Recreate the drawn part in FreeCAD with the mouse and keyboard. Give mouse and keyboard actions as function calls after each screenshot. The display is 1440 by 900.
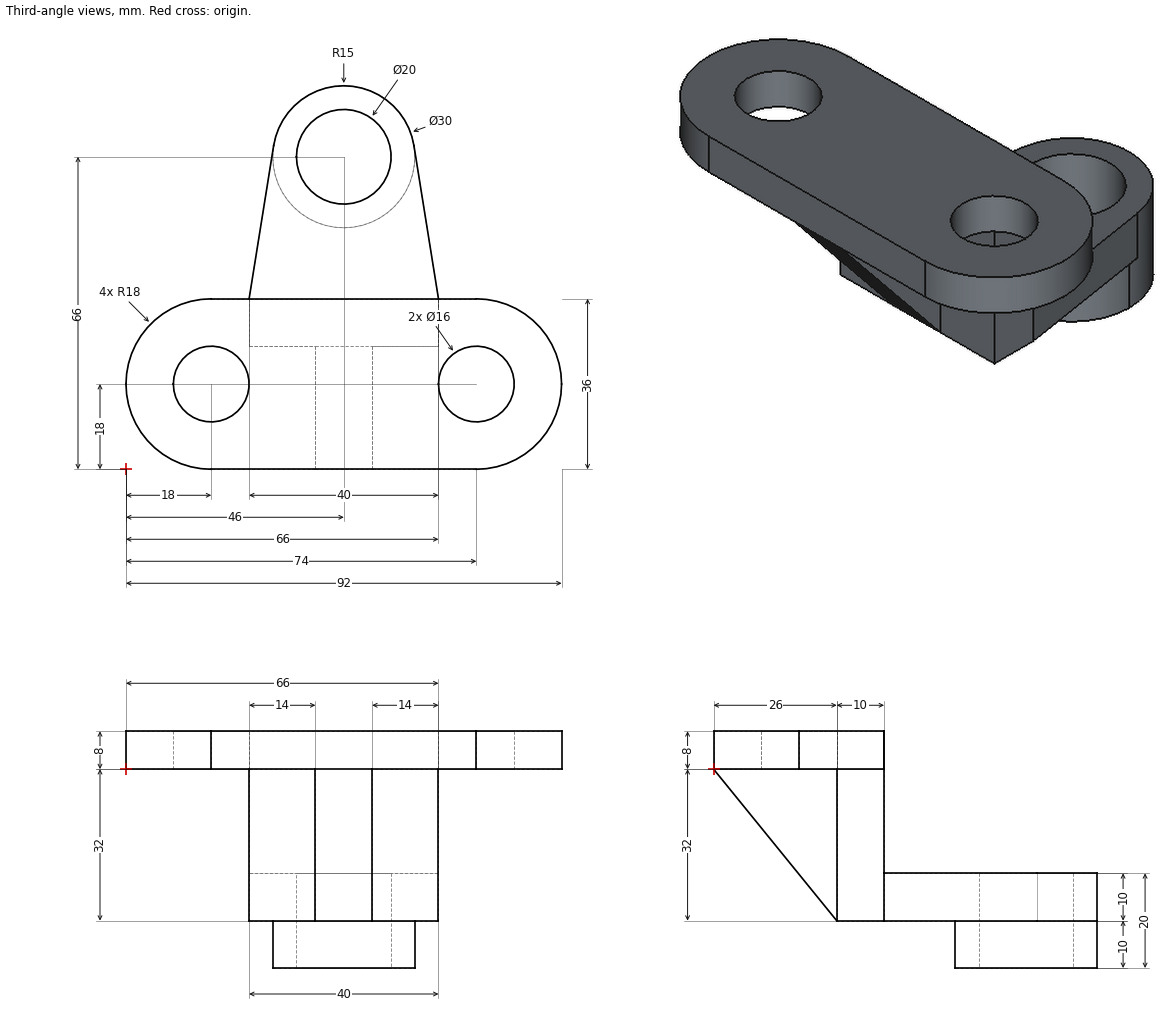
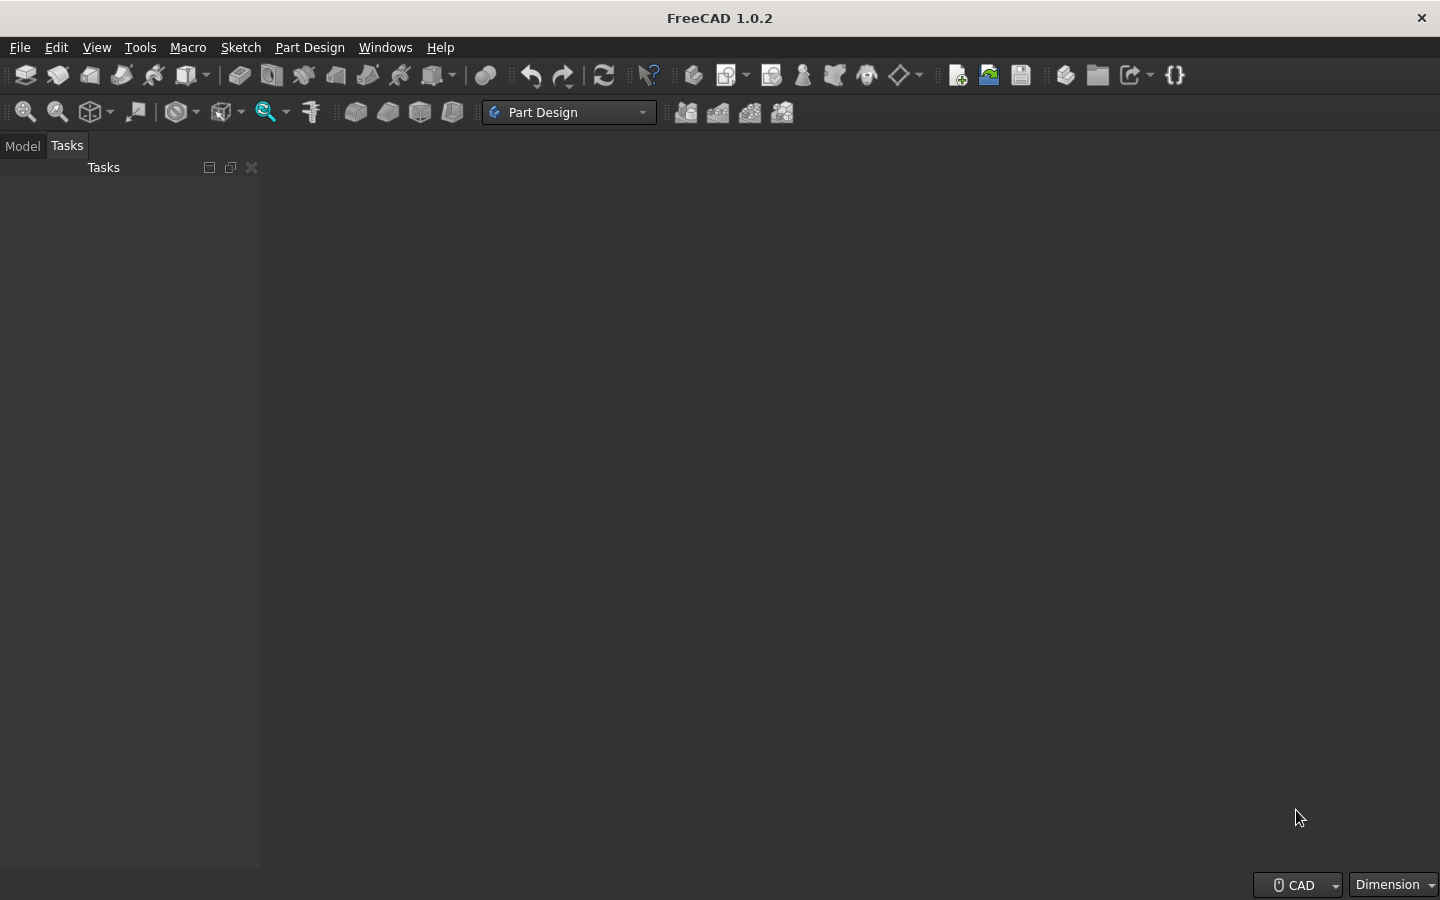
click(958, 76)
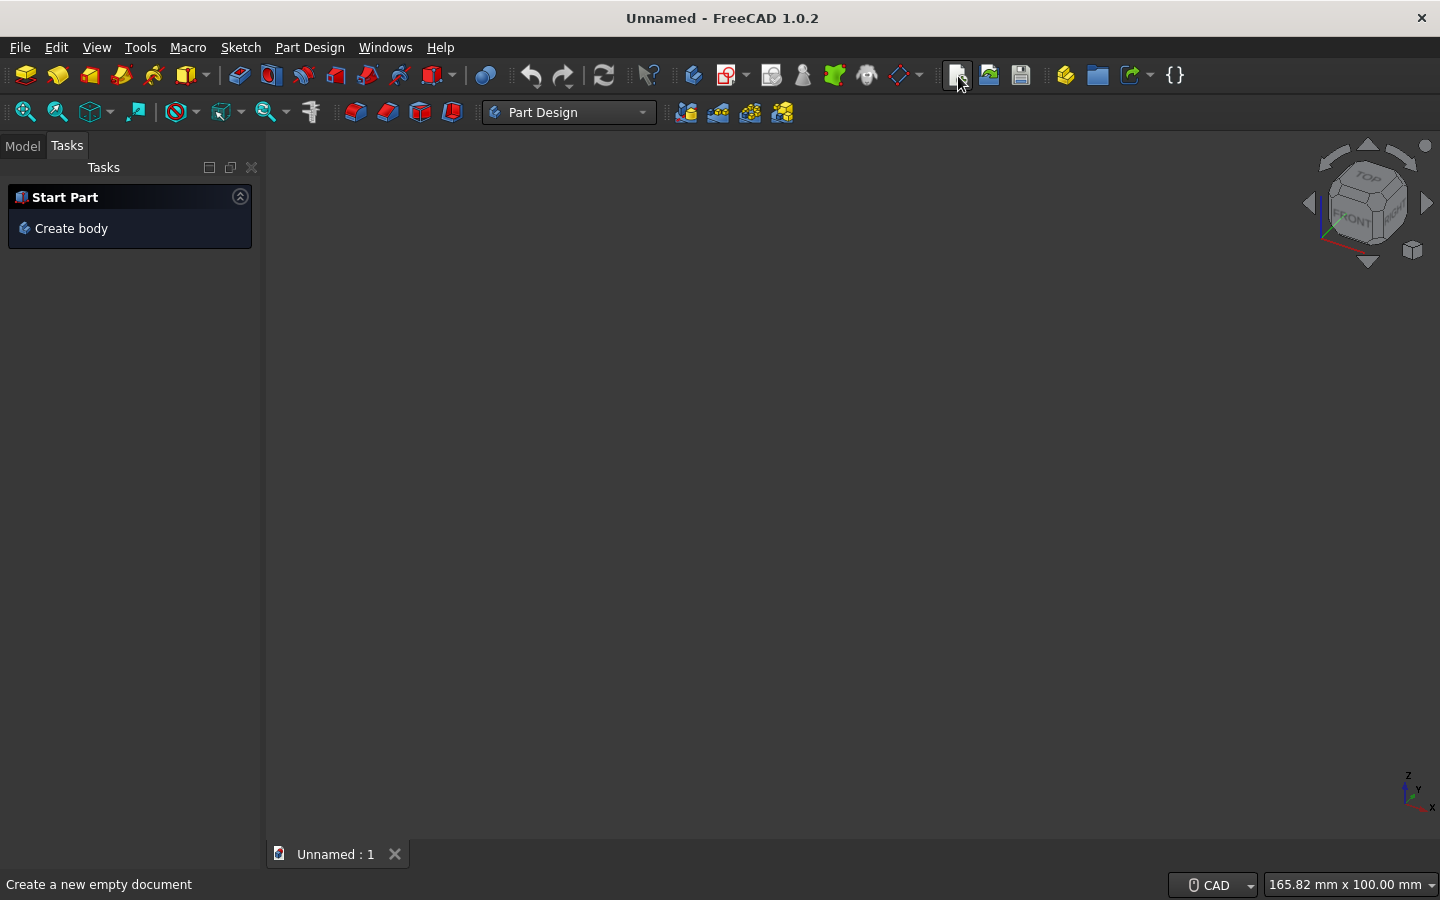
click(726, 76)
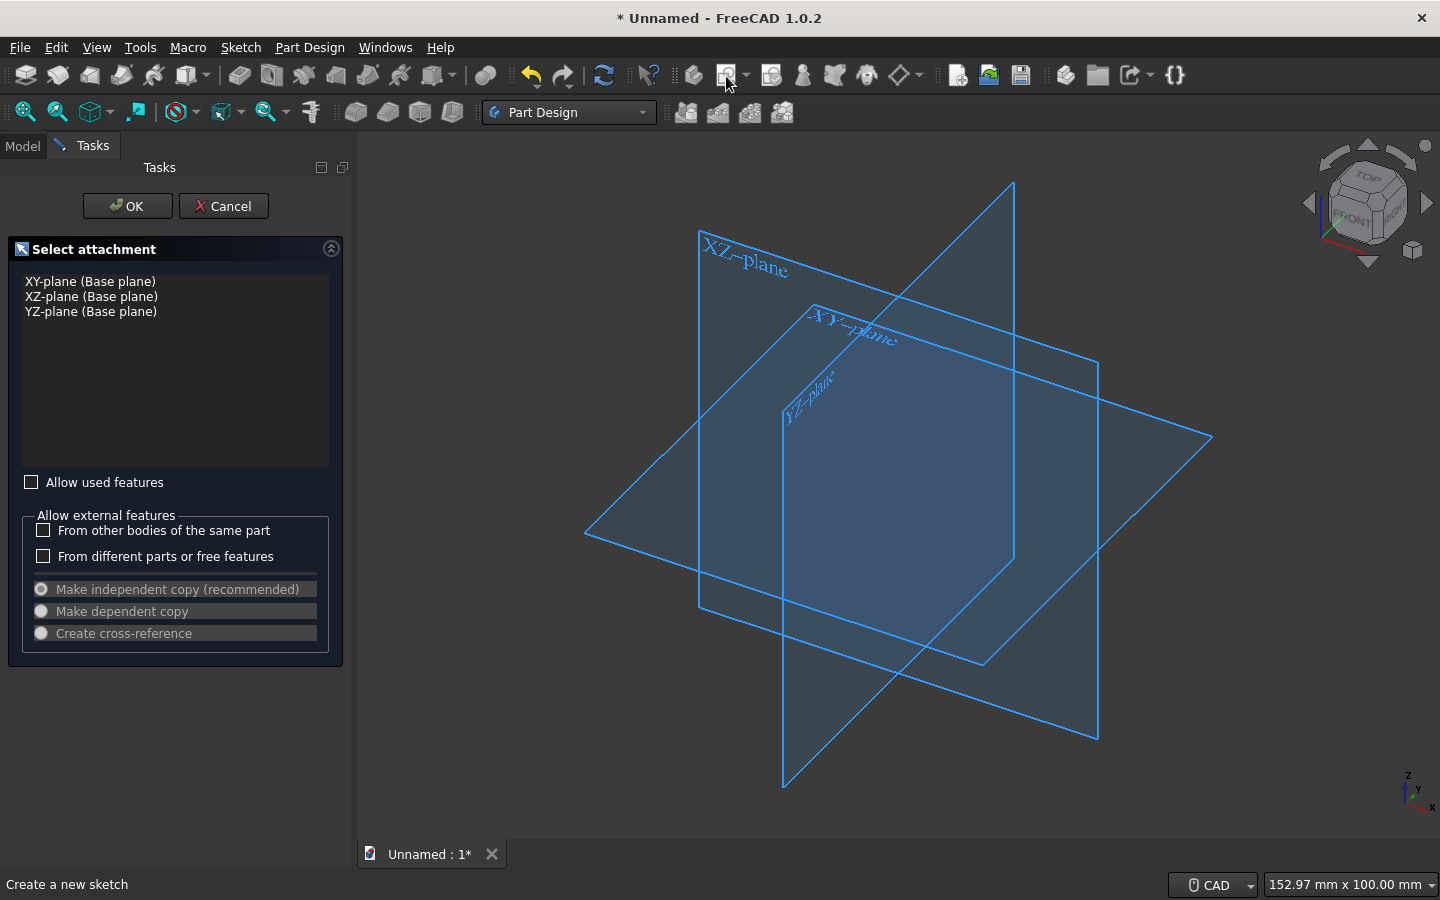
click(82, 282)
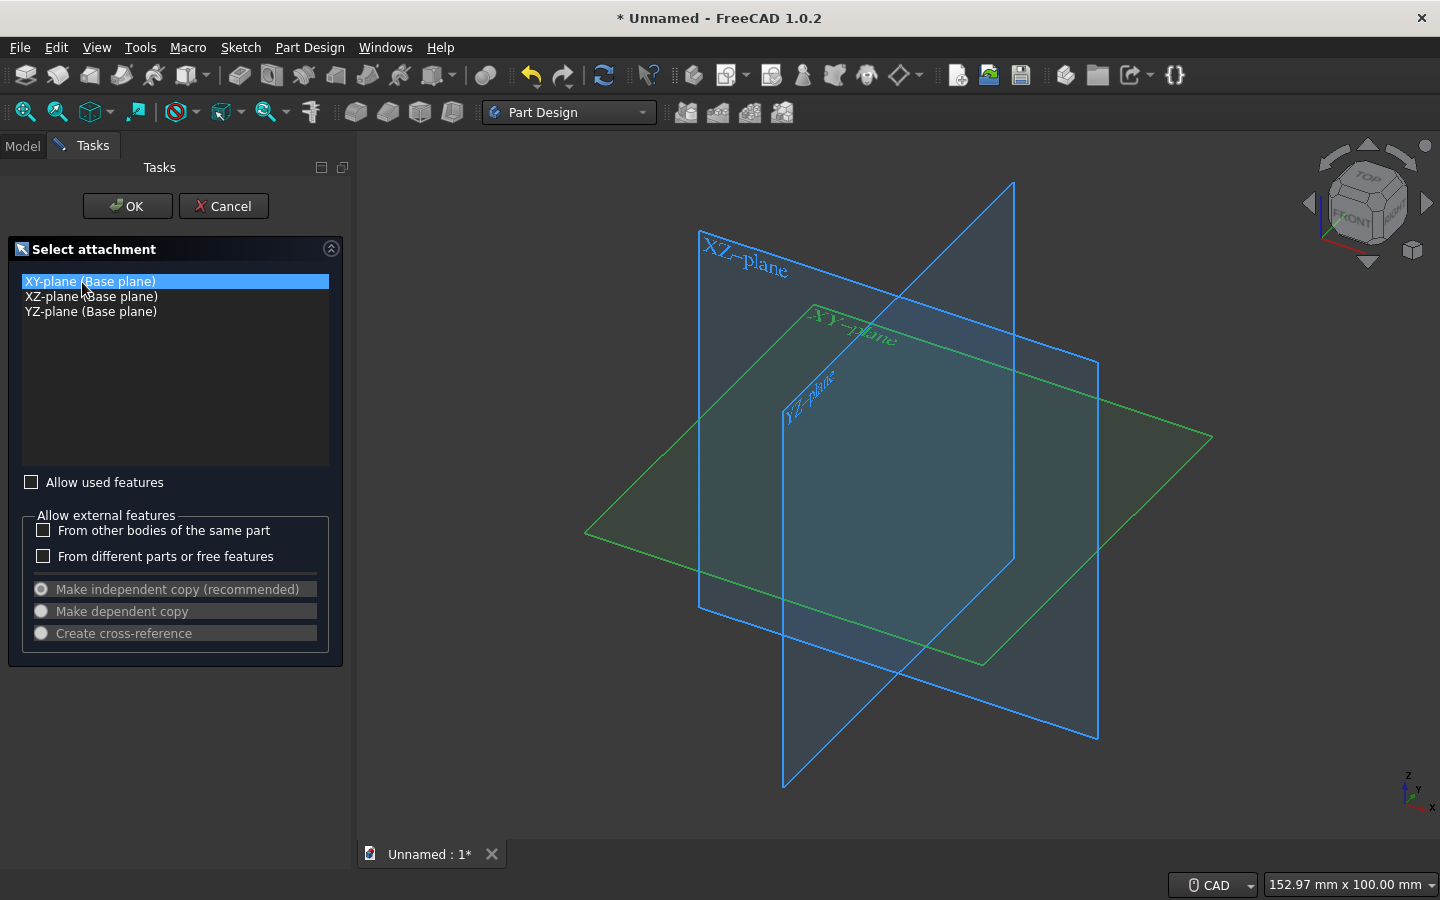
click(128, 206)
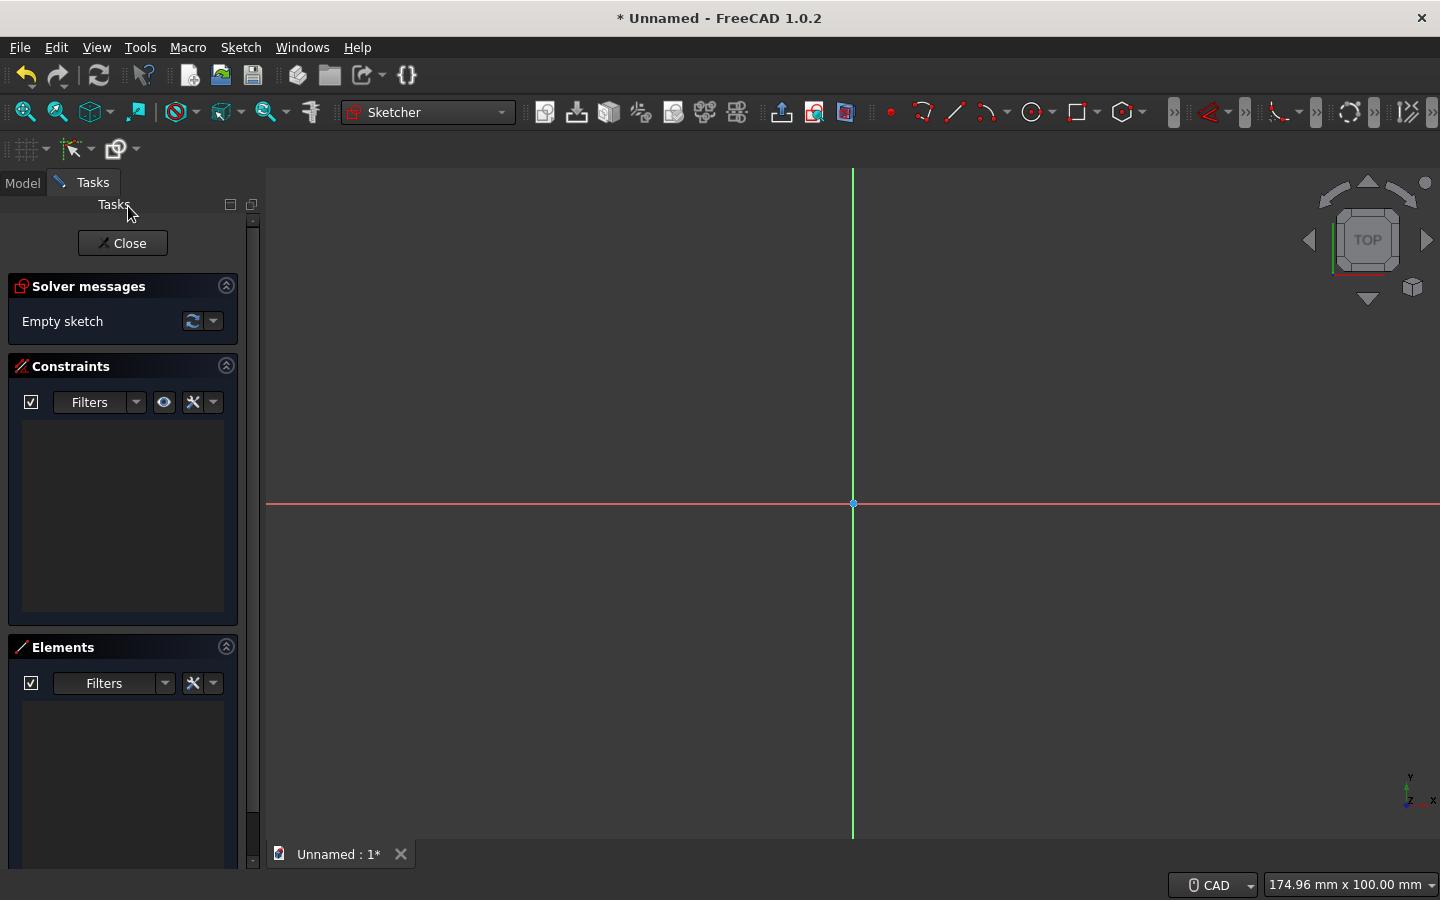
scroll(294, 749, down, 2)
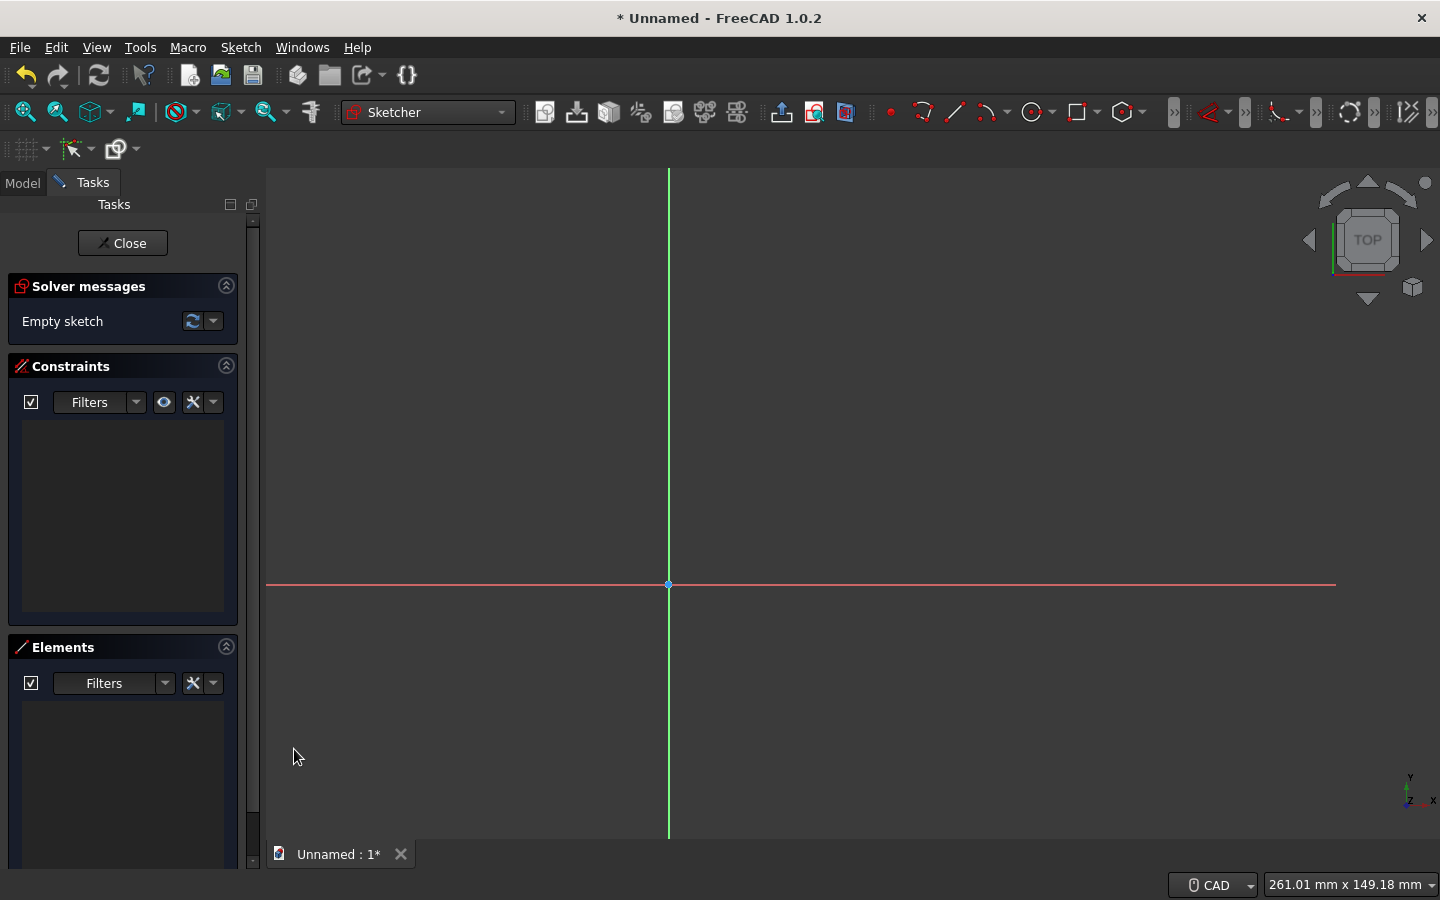
scroll(986, 504, up, 3)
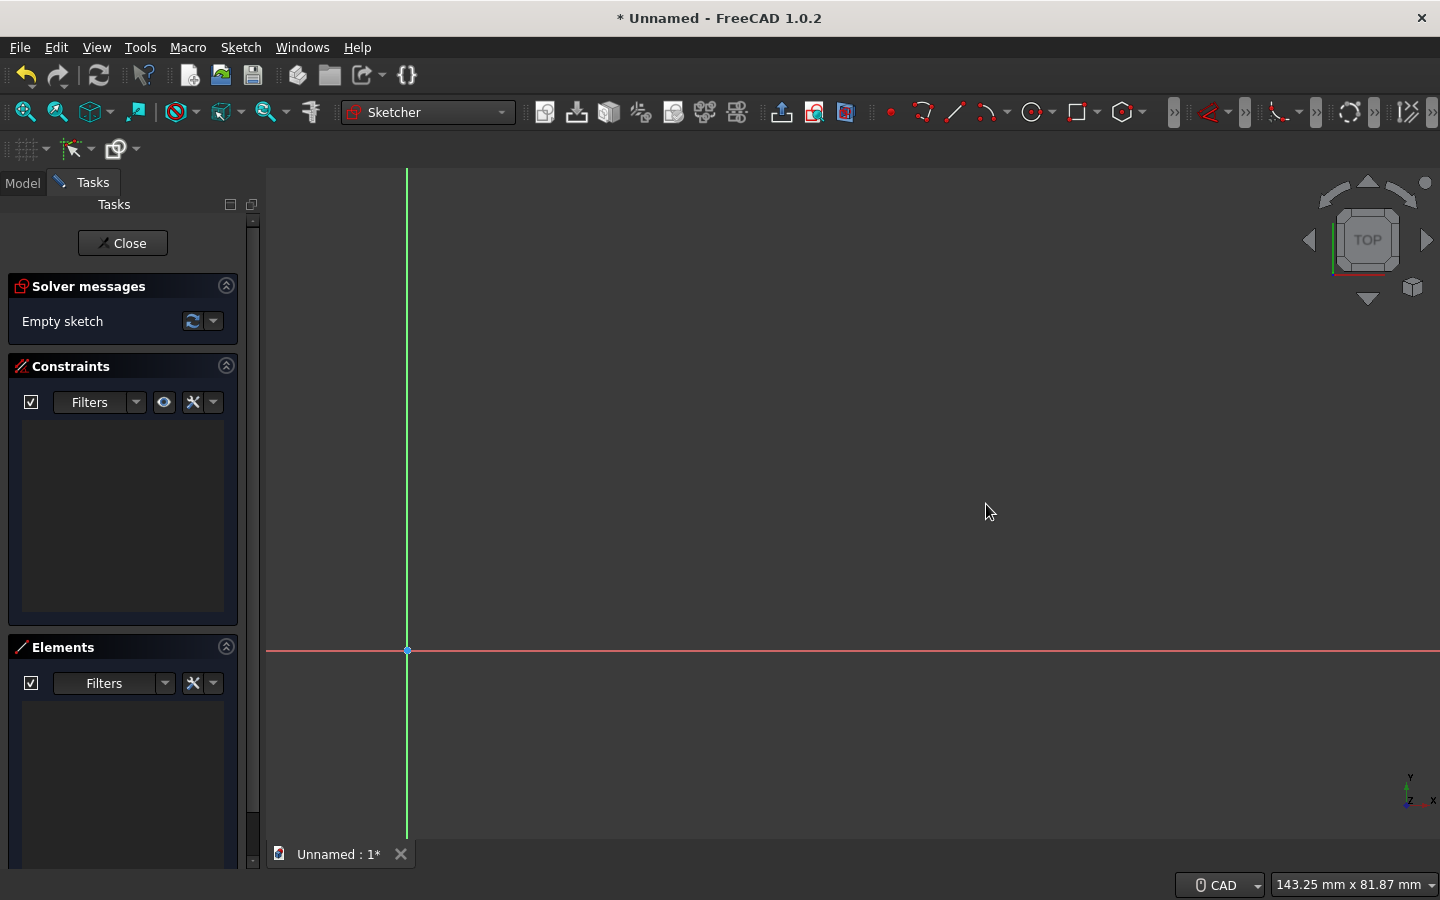
click(1078, 112)